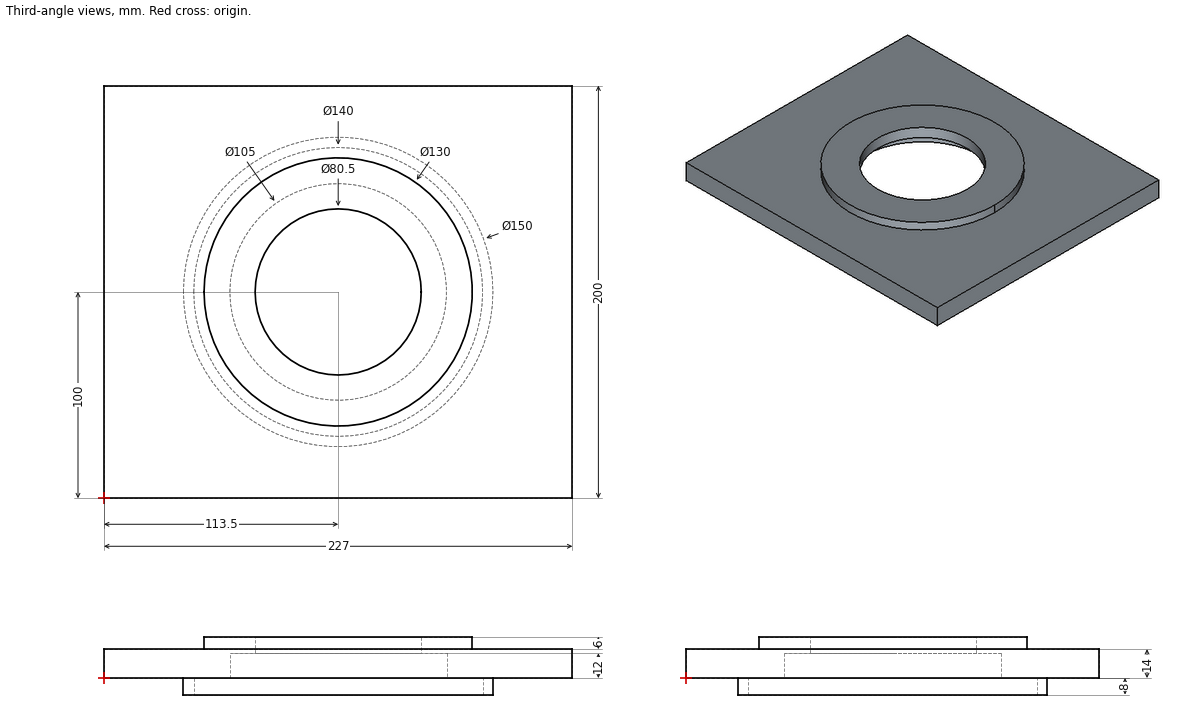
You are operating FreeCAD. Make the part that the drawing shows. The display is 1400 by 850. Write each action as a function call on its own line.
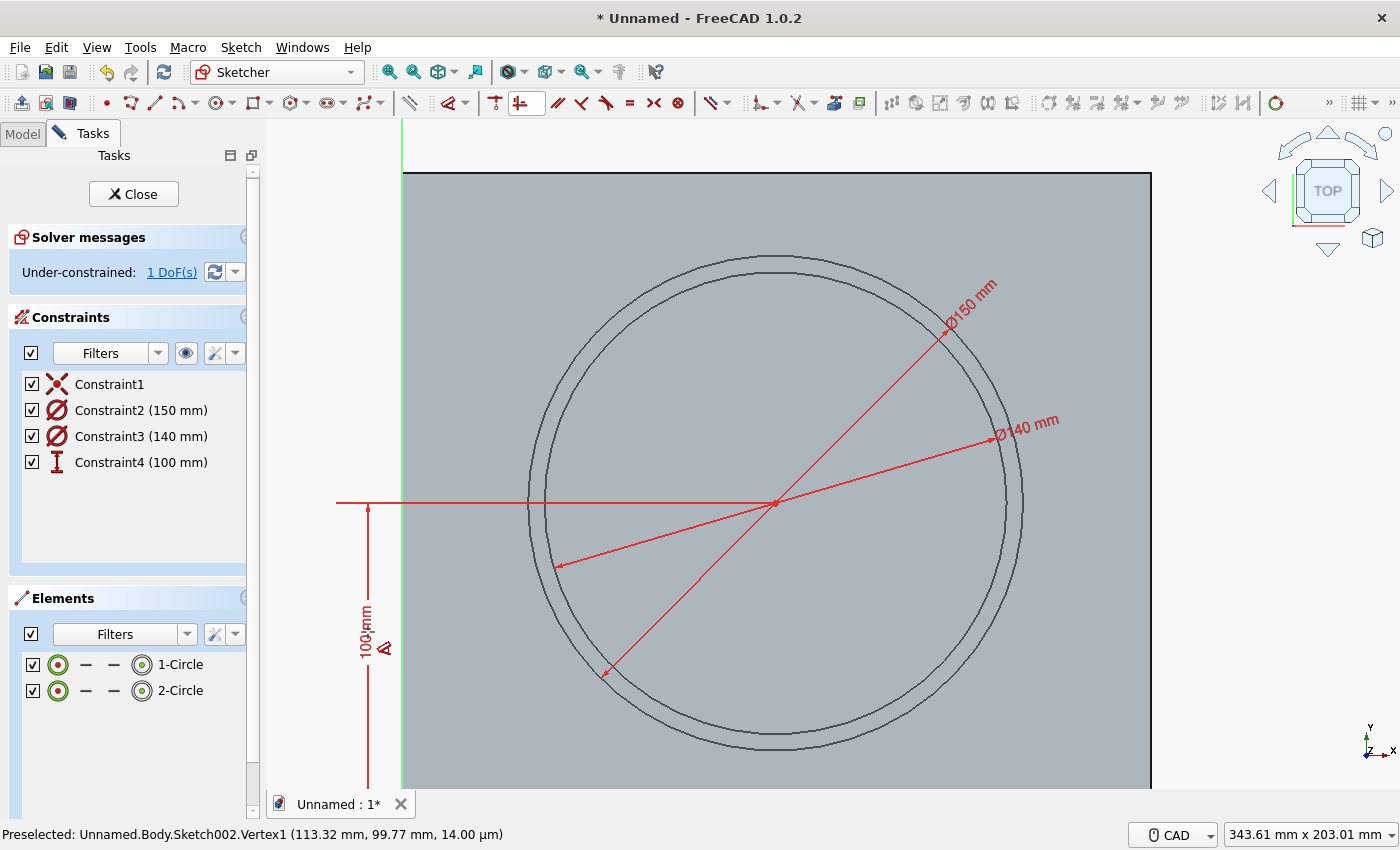
click(776, 503)
click(589, 469)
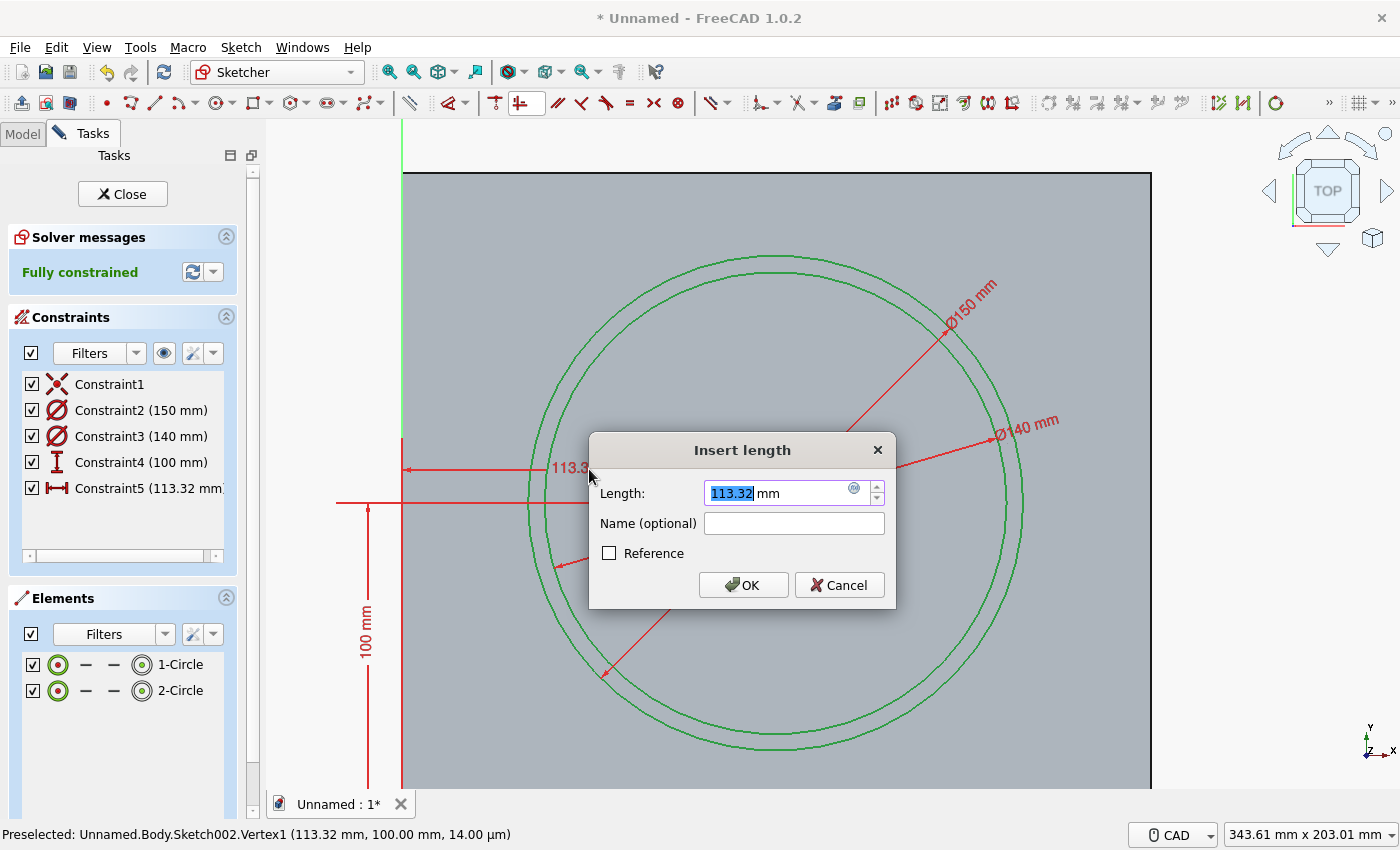
text(113.5)
key(Return)
key(Escape)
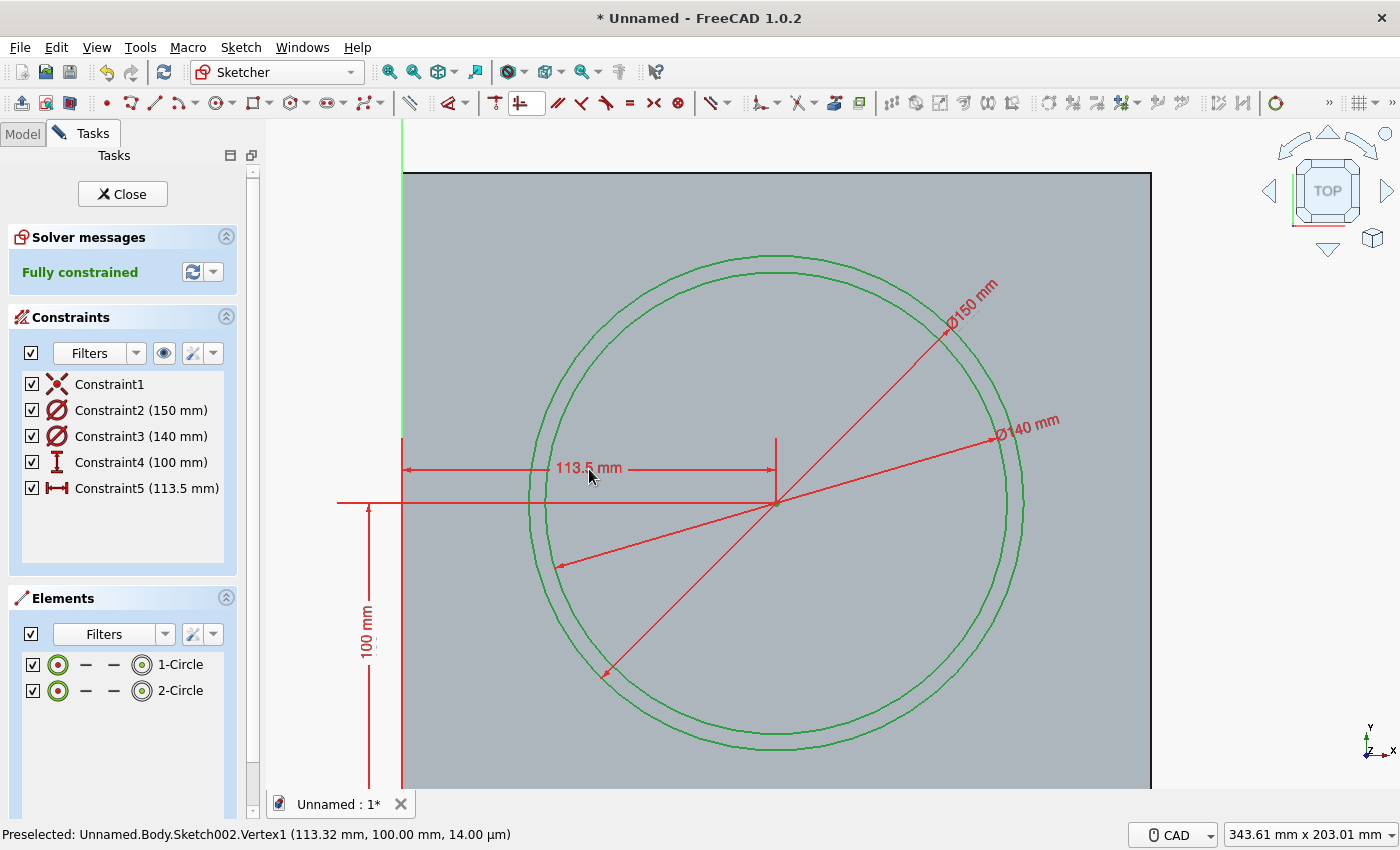
click(123, 194)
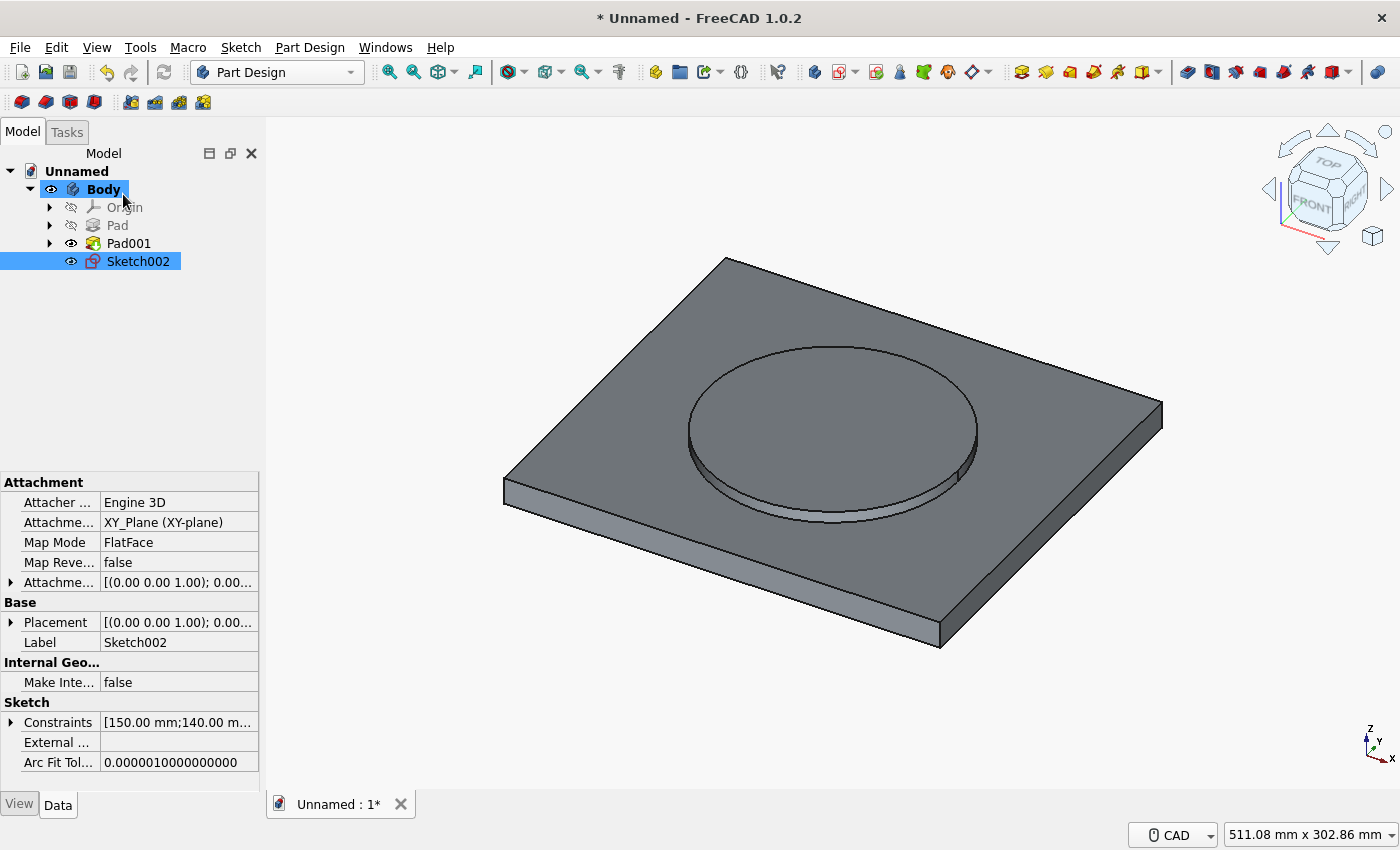
click(1022, 72)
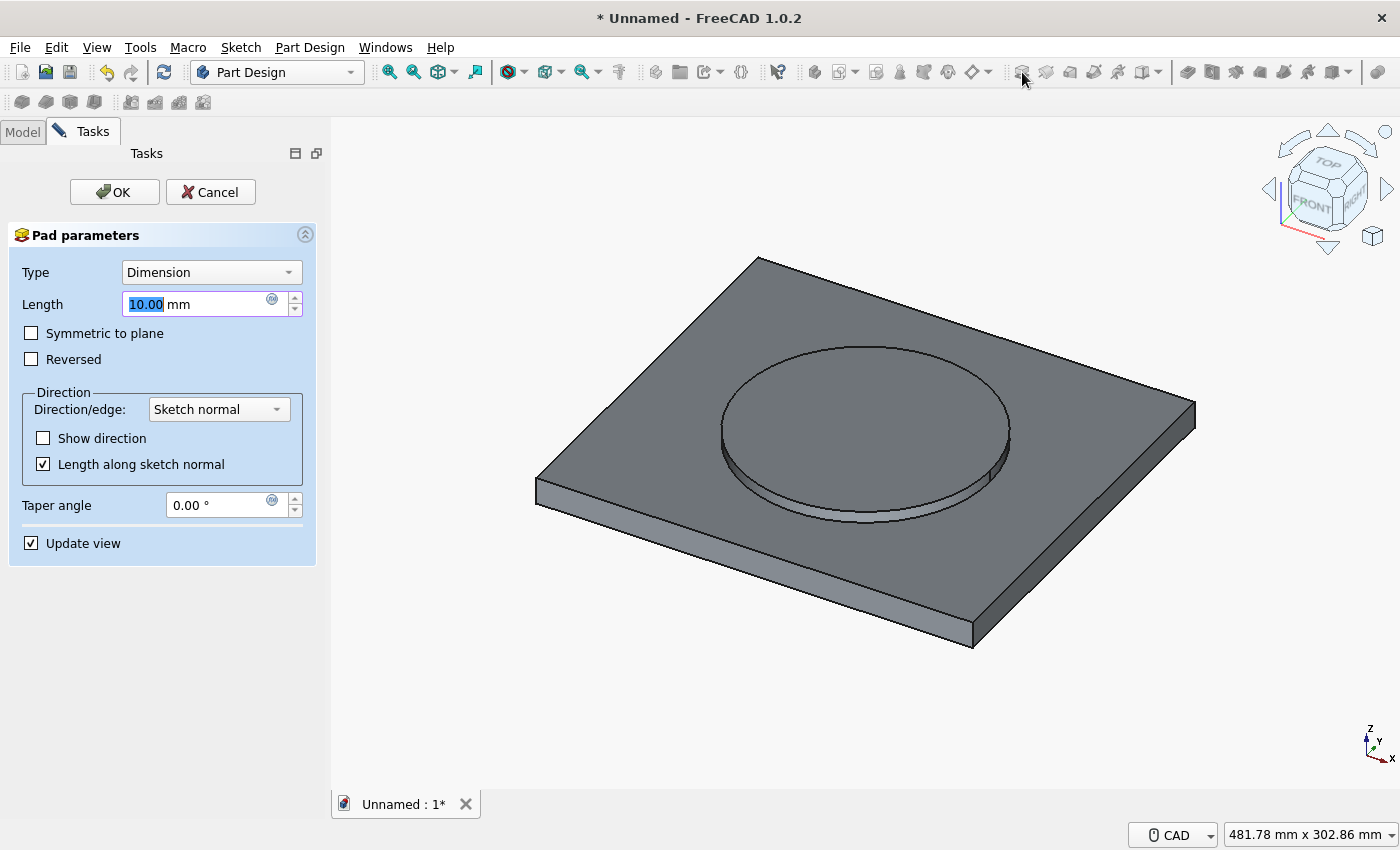
text(8)
key(Tab)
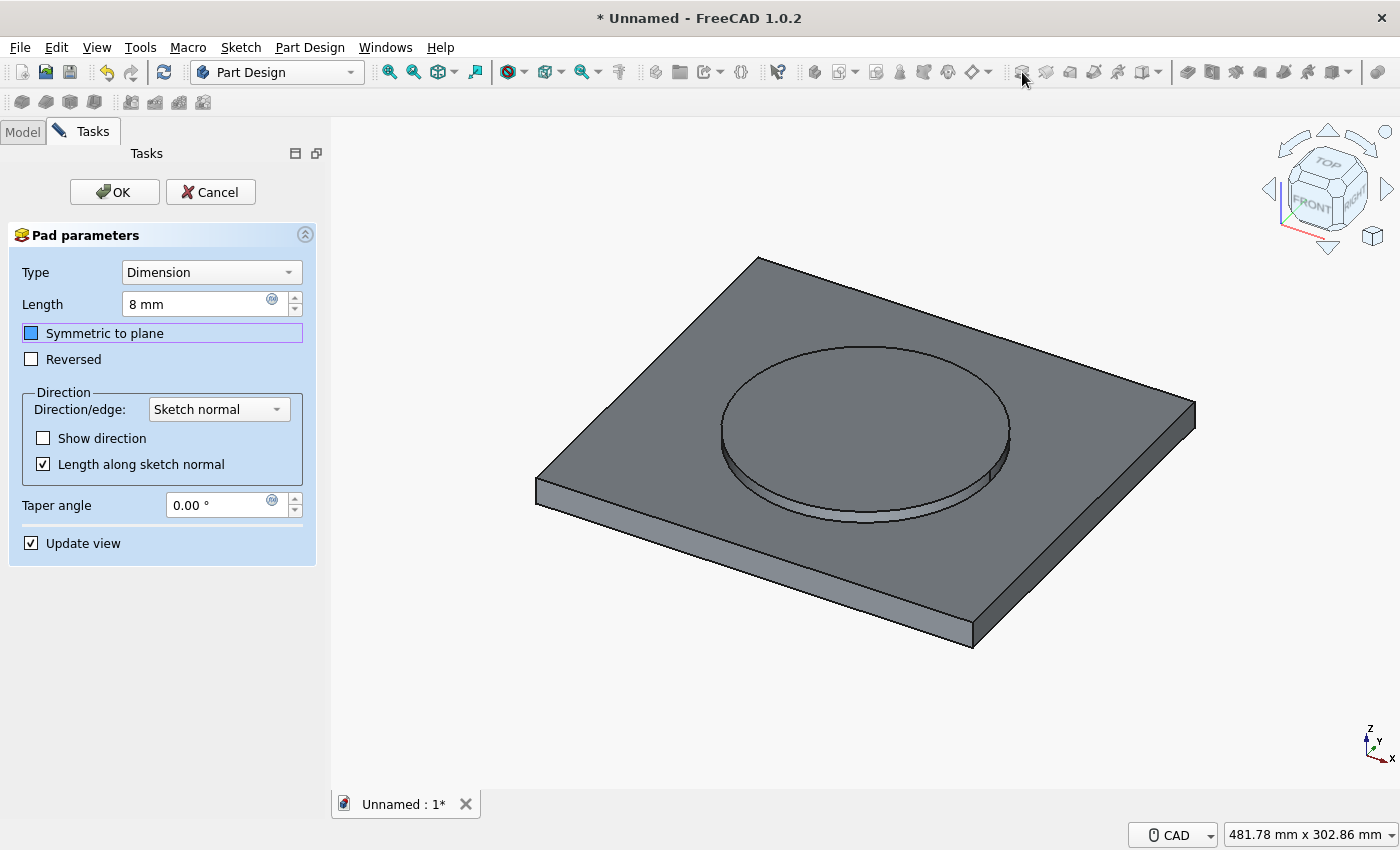
click(30, 359)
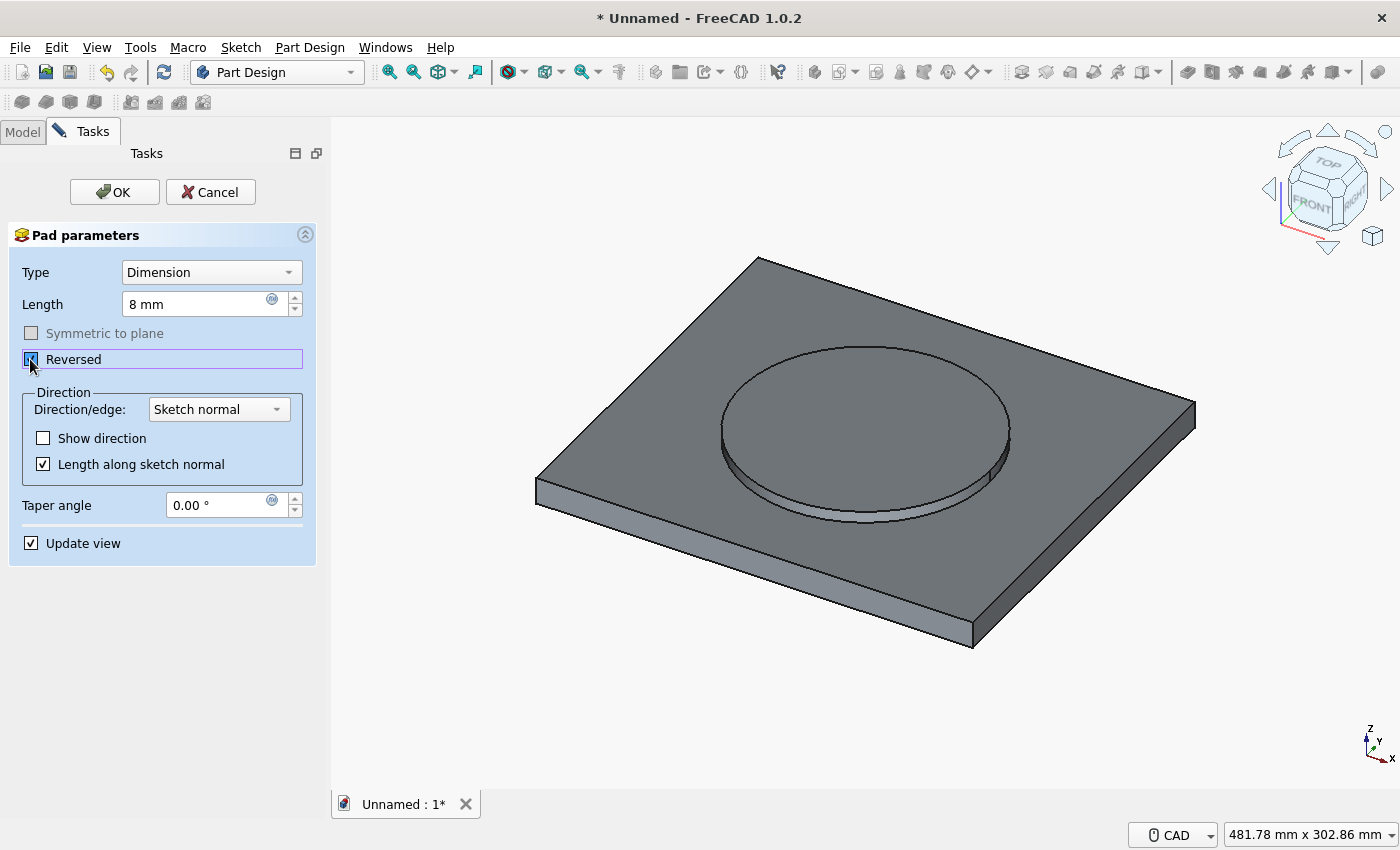
click(115, 192)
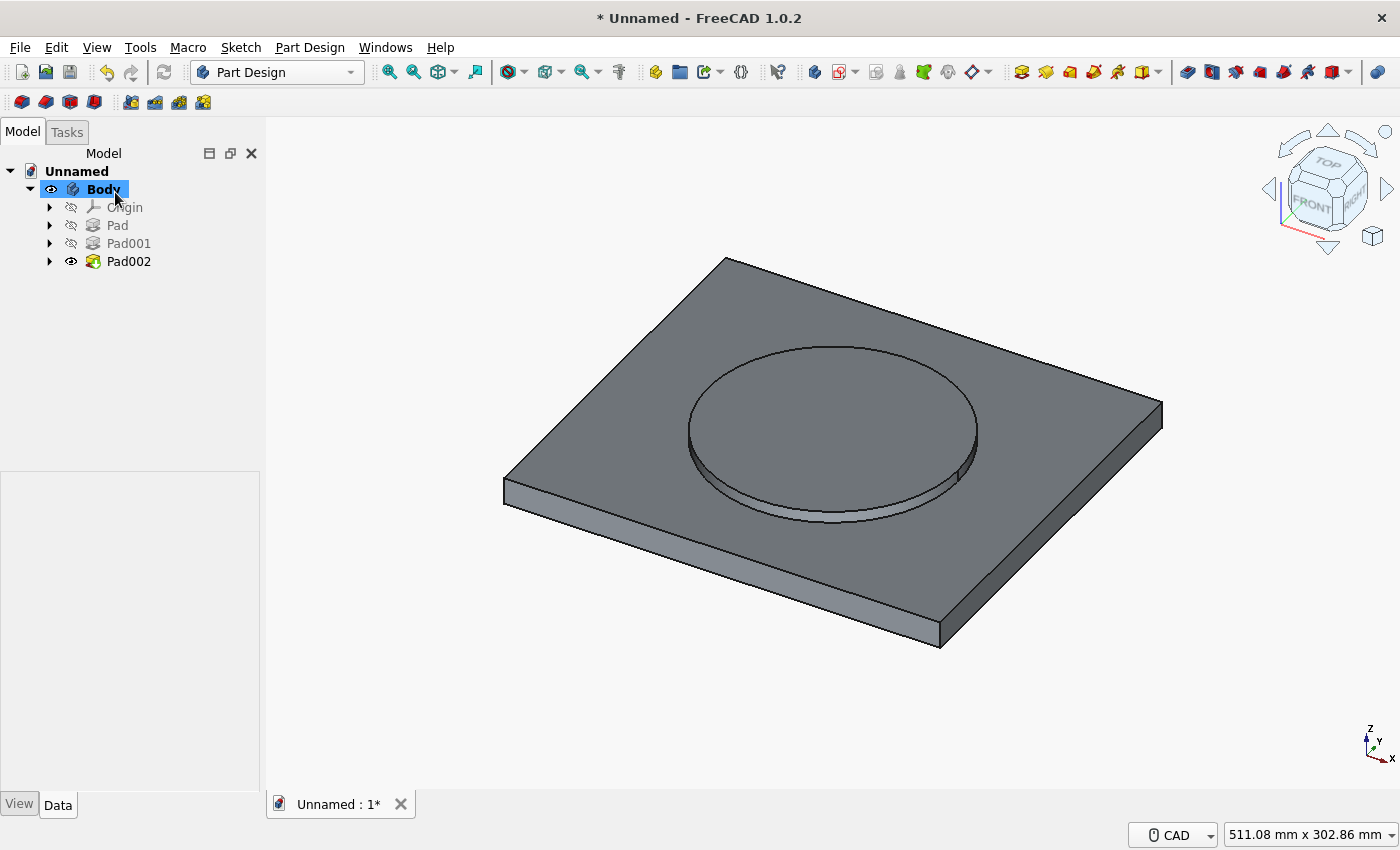
click(833, 428)